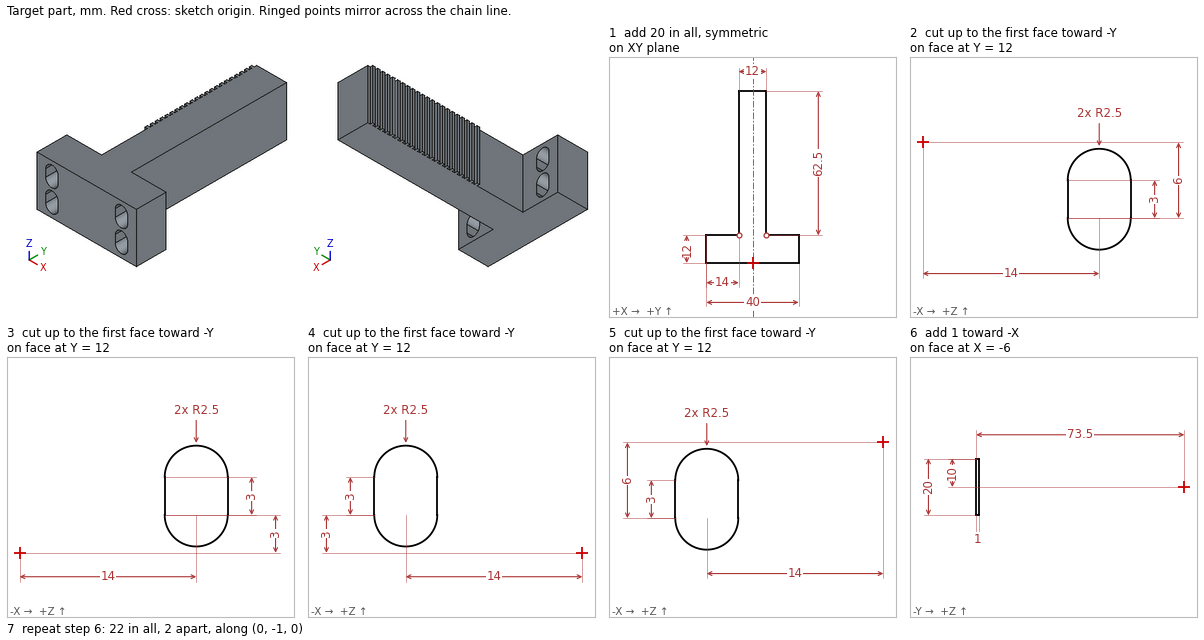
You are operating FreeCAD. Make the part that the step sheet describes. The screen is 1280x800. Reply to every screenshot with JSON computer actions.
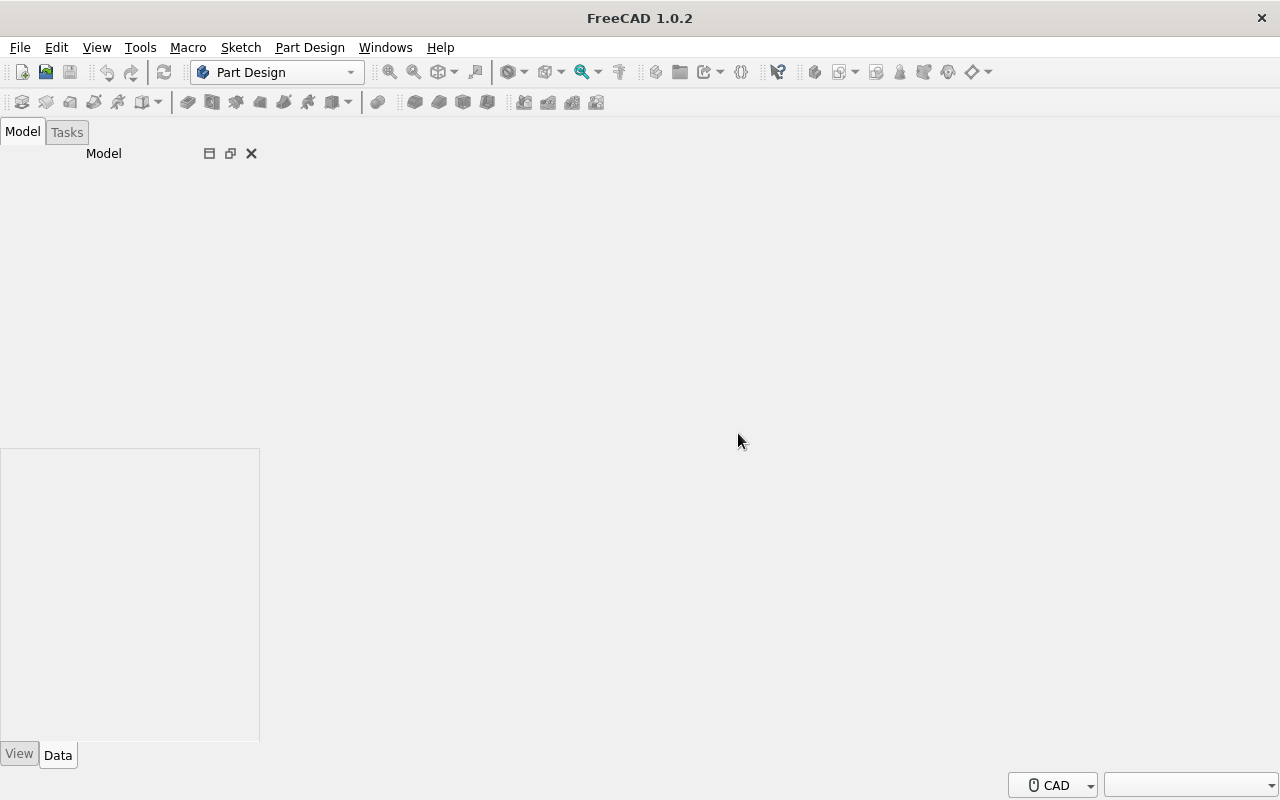
{"action": "left_click", "coordinate": [22, 72]}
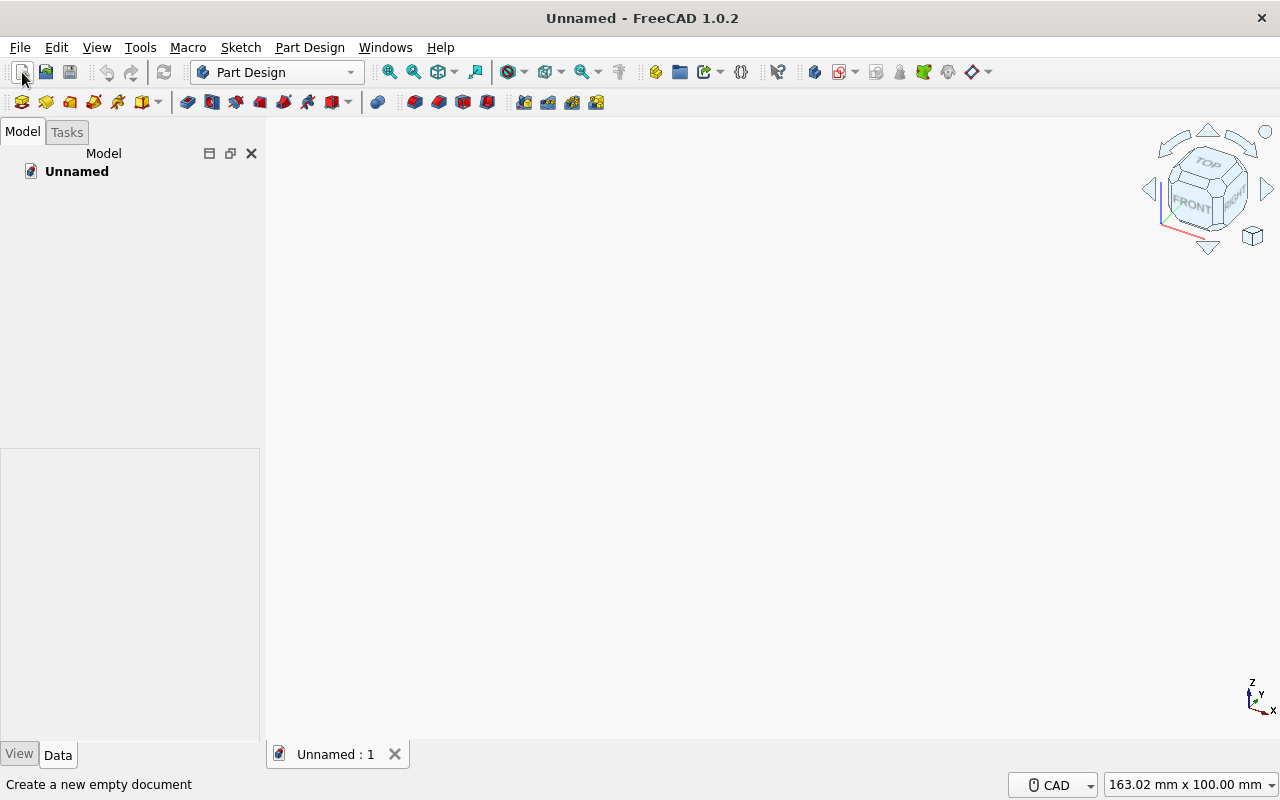
{"action": "left_click", "coordinate": [840, 72]}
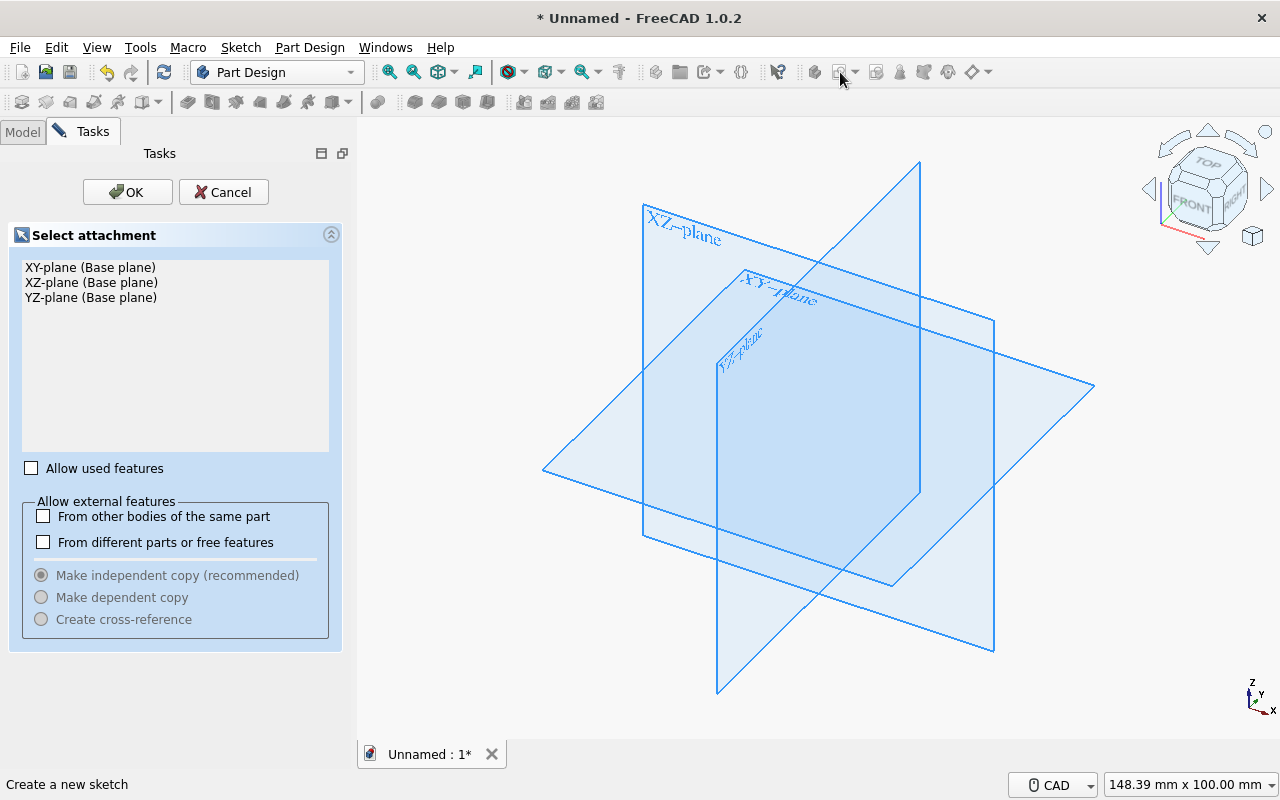
{"action": "left_click", "coordinate": [82, 268]}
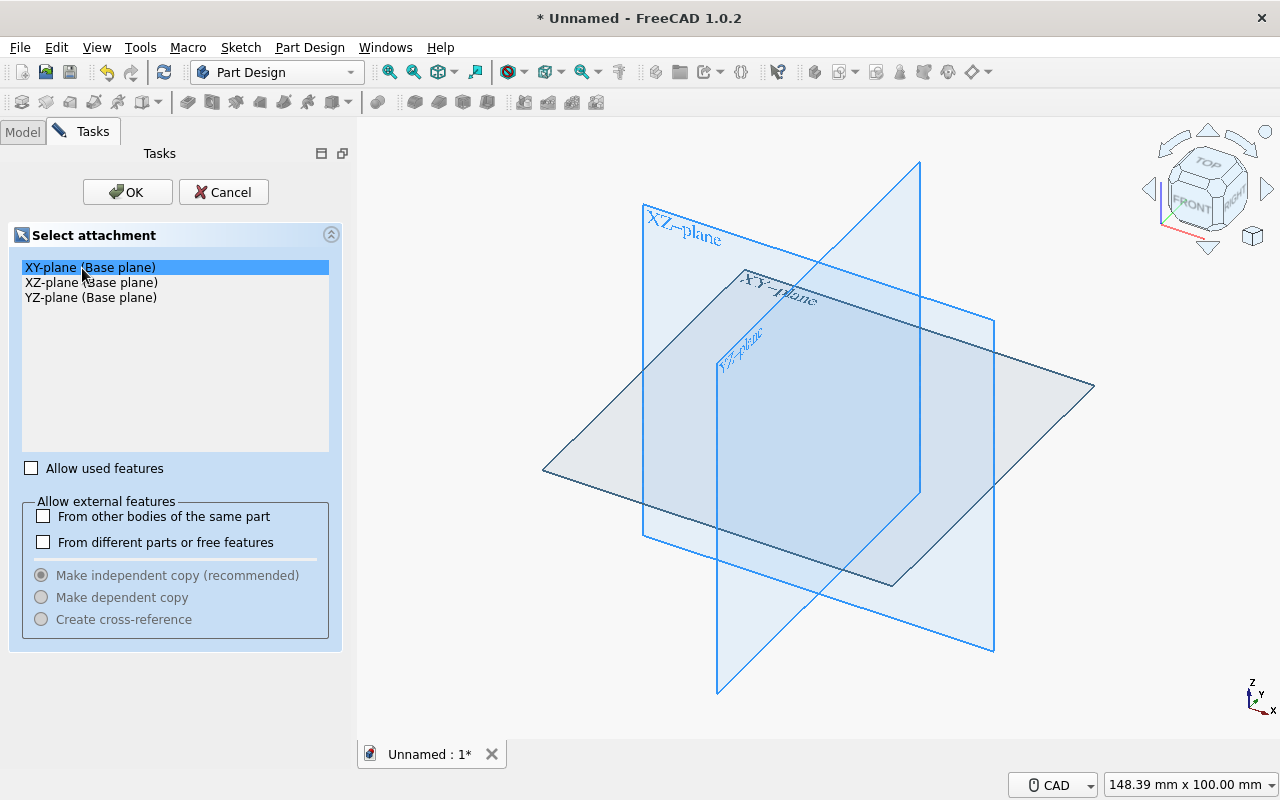
{"action": "left_click", "coordinate": [128, 192]}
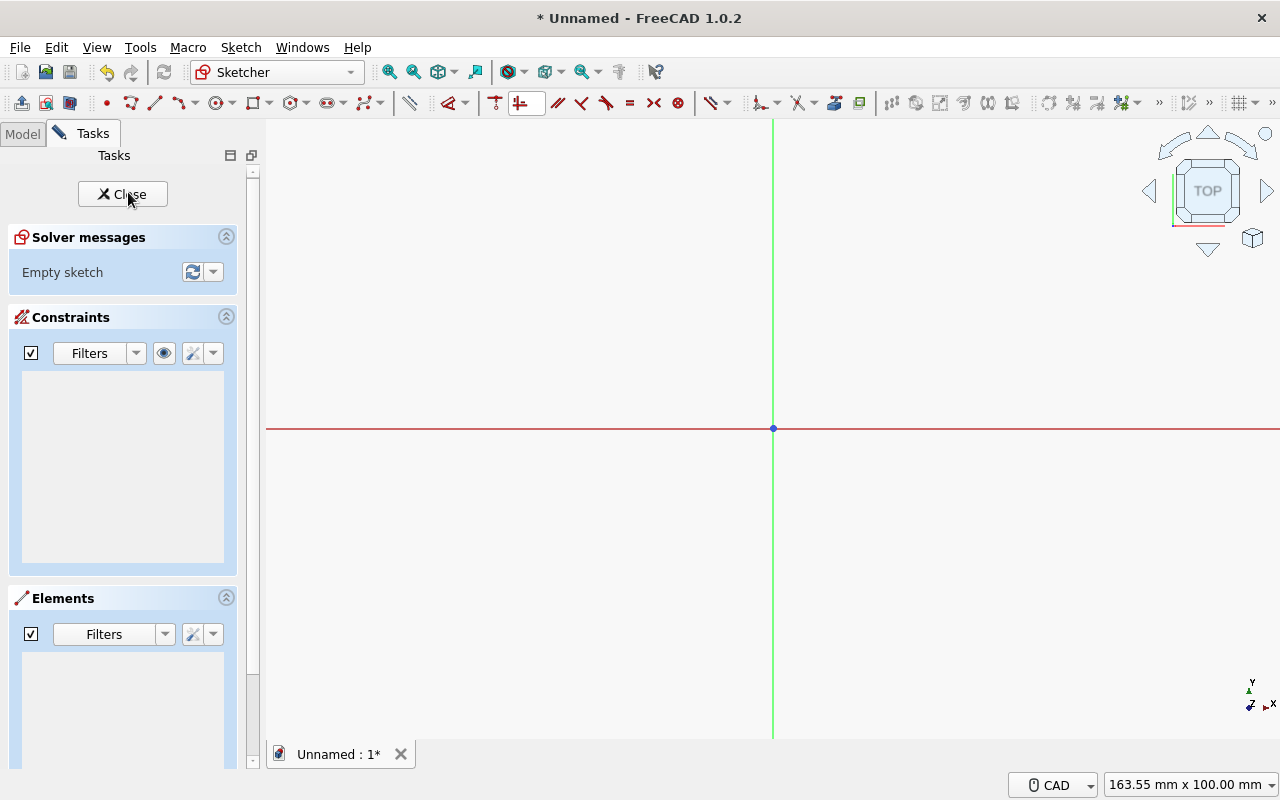
{"action": "scroll", "coordinate": [565, 711], "scroll_direction": "down", "scroll_amount": 2}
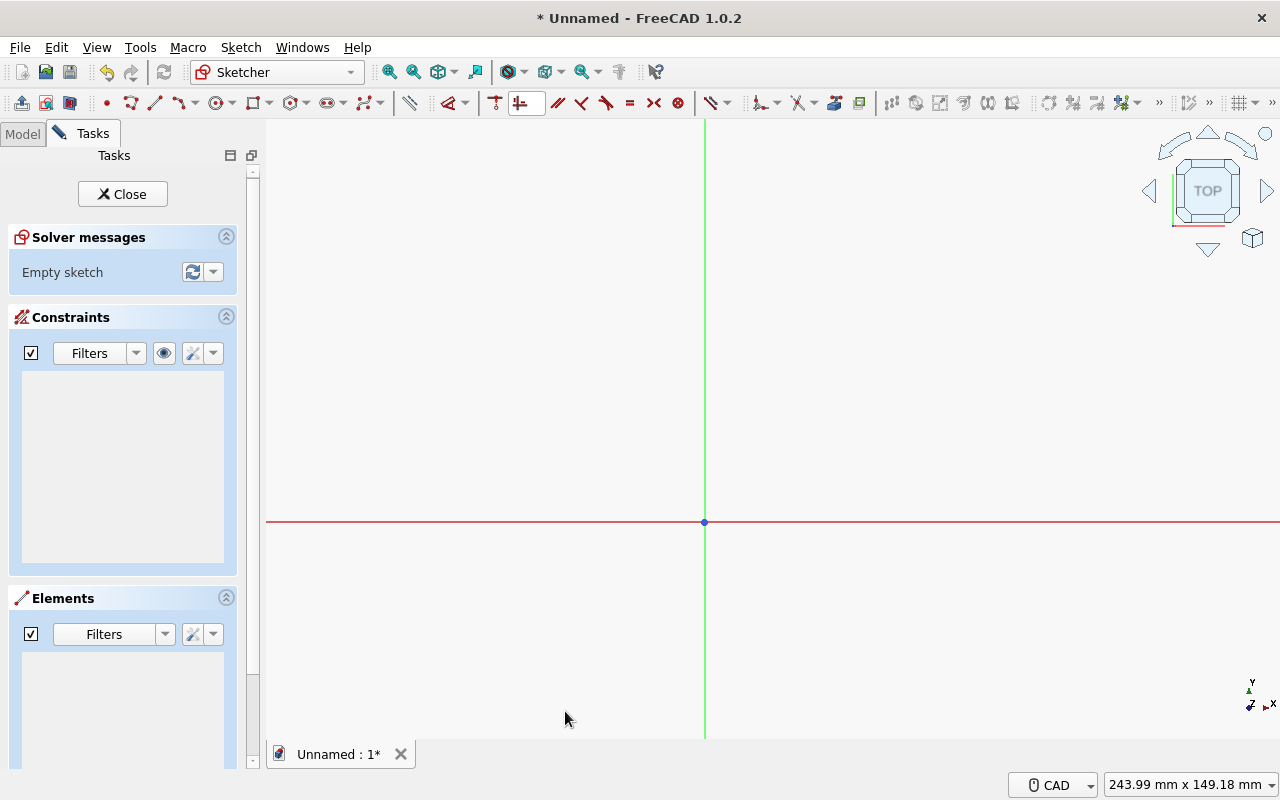
{"action": "left_click", "coordinate": [132, 104]}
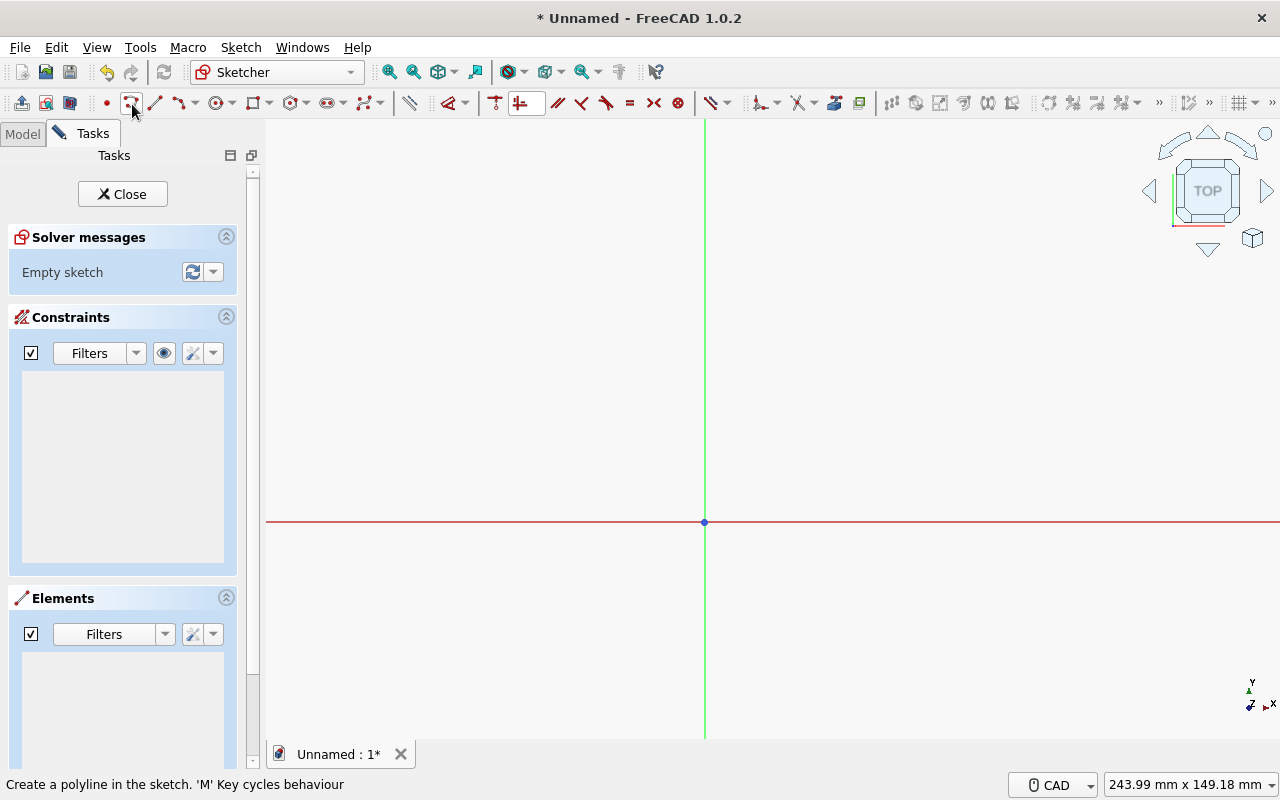
{"action": "left_click", "coordinate": [729, 472]}
{"action": "left_click", "coordinate": [729, 213]}
{"action": "left_click", "coordinate": [680, 213]}
{"action": "left_click", "coordinate": [680, 472]}
{"action": "left_click", "coordinate": [621, 472]}
{"action": "left_click", "coordinate": [621, 522]}
{"action": "left_click", "coordinate": [788, 513]}
{"action": "left_click", "coordinate": [788, 472]}
{"action": "left_click", "coordinate": [729, 473]}
{"action": "key", "text": "Escape"}
{"action": "key", "text": "Escape"}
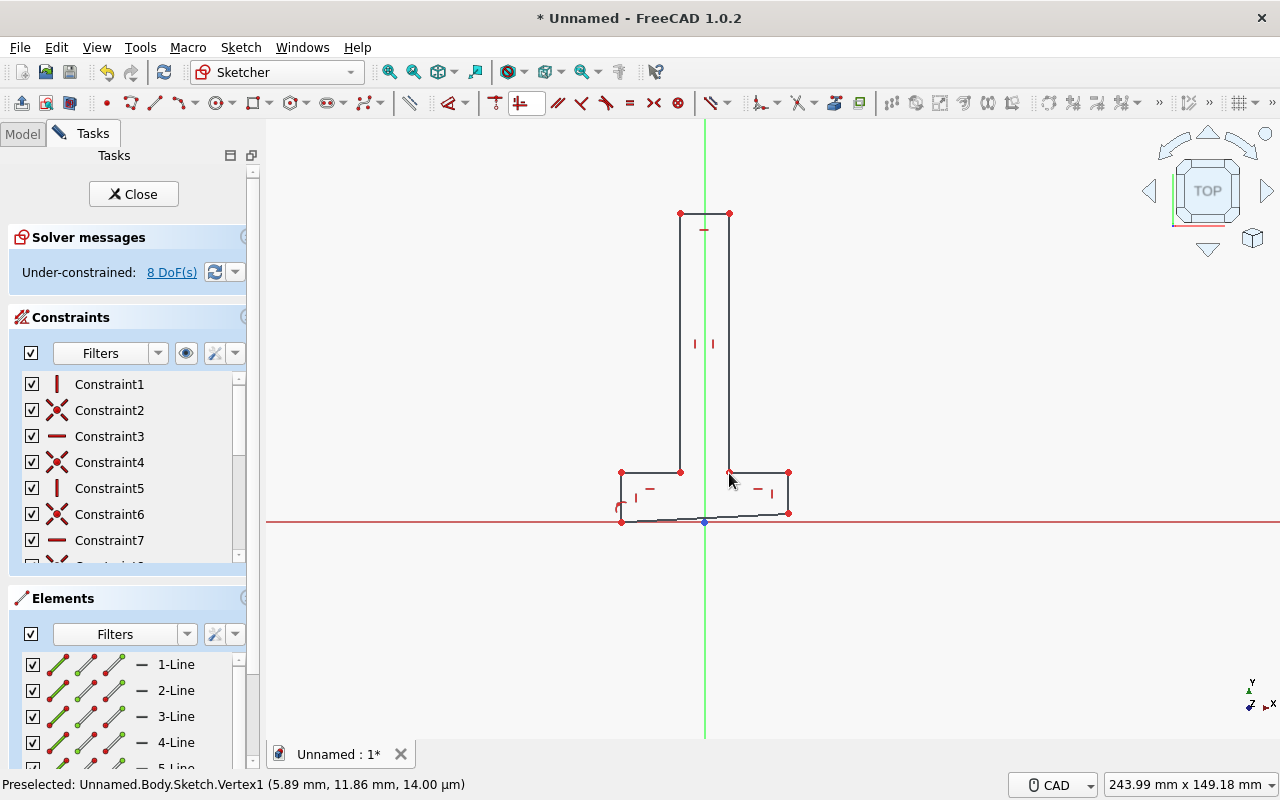
{"action": "left_click", "coordinate": [671, 520]}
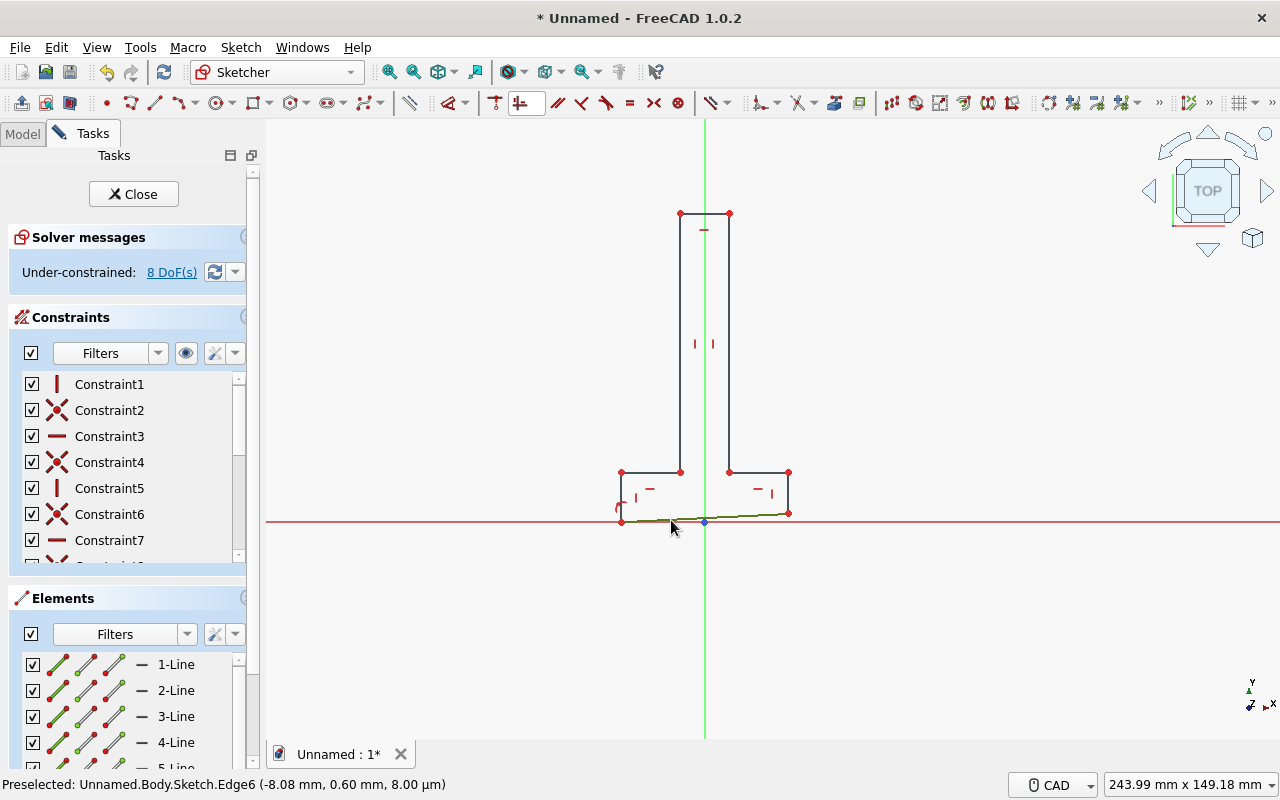
{"action": "left_click", "coordinate": [540, 104]}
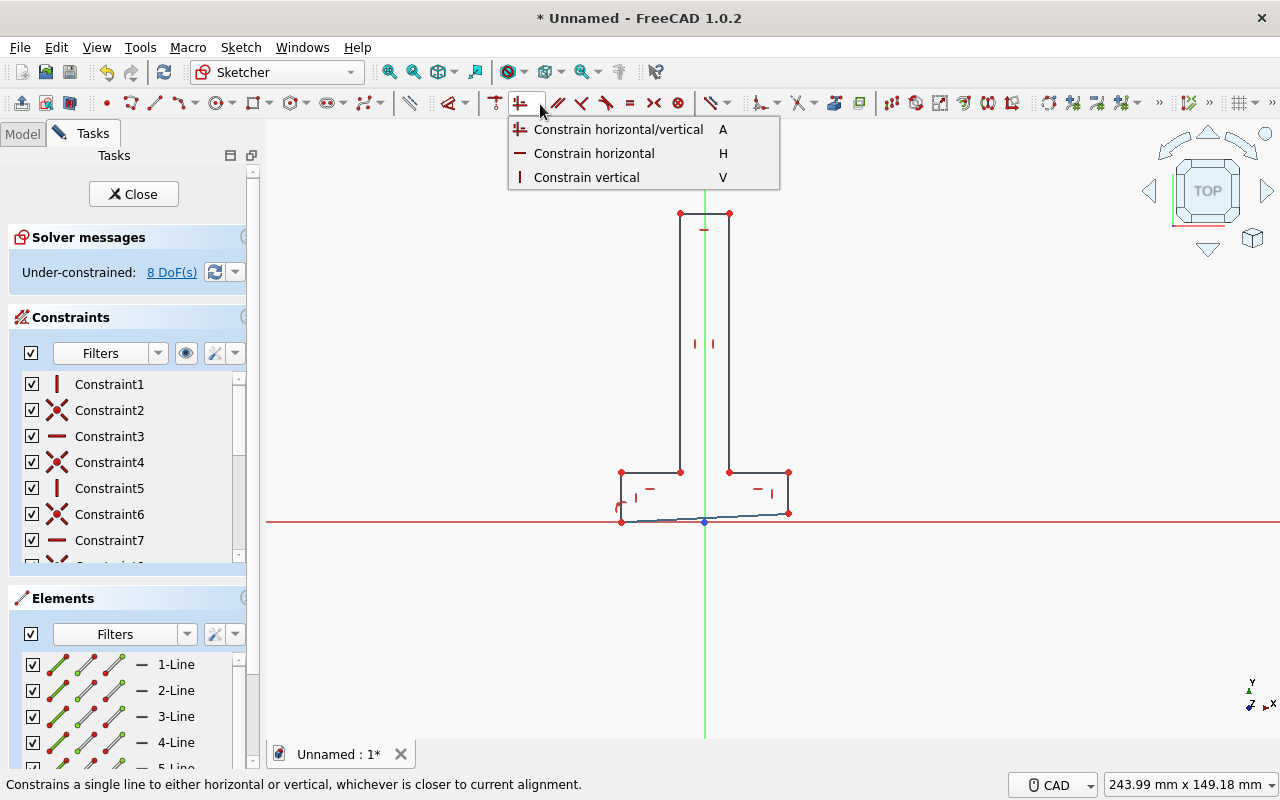
{"action": "left_click", "coordinate": [644, 153]}